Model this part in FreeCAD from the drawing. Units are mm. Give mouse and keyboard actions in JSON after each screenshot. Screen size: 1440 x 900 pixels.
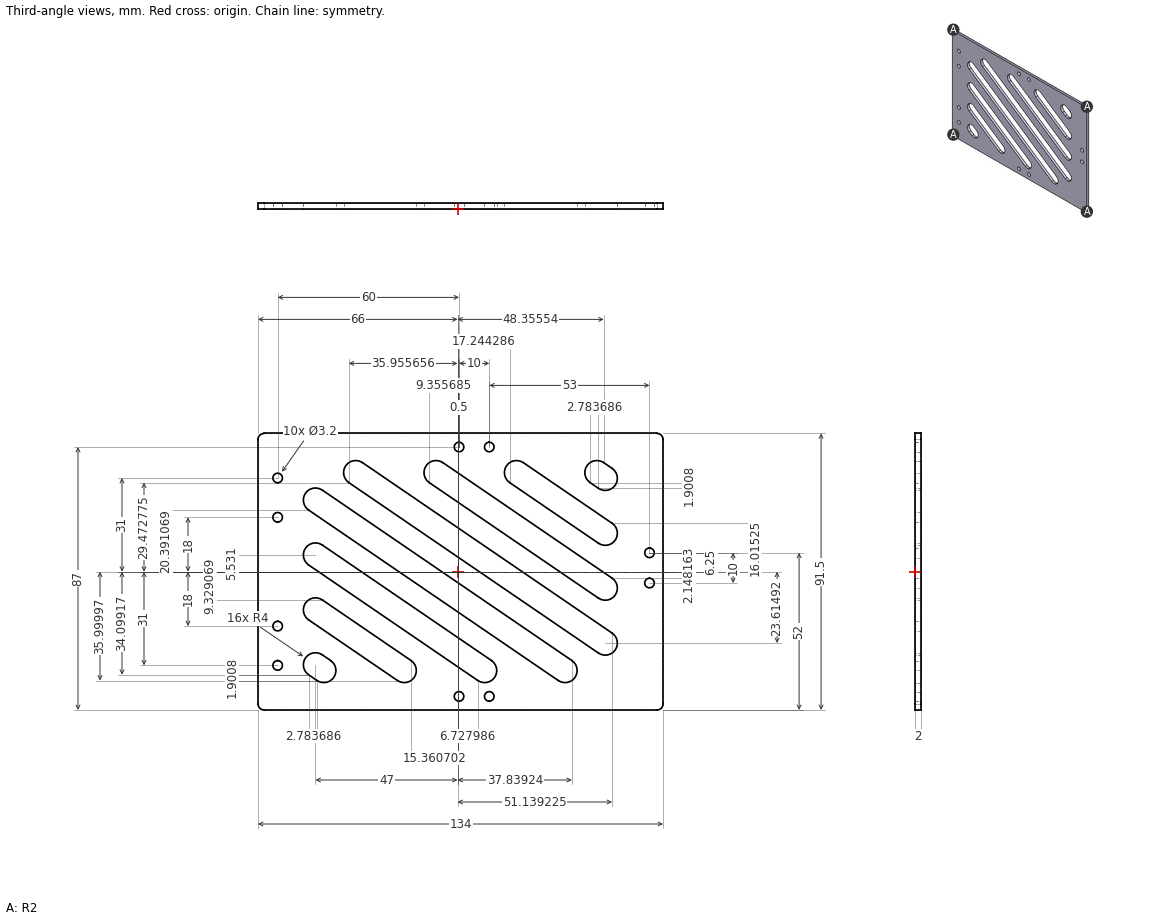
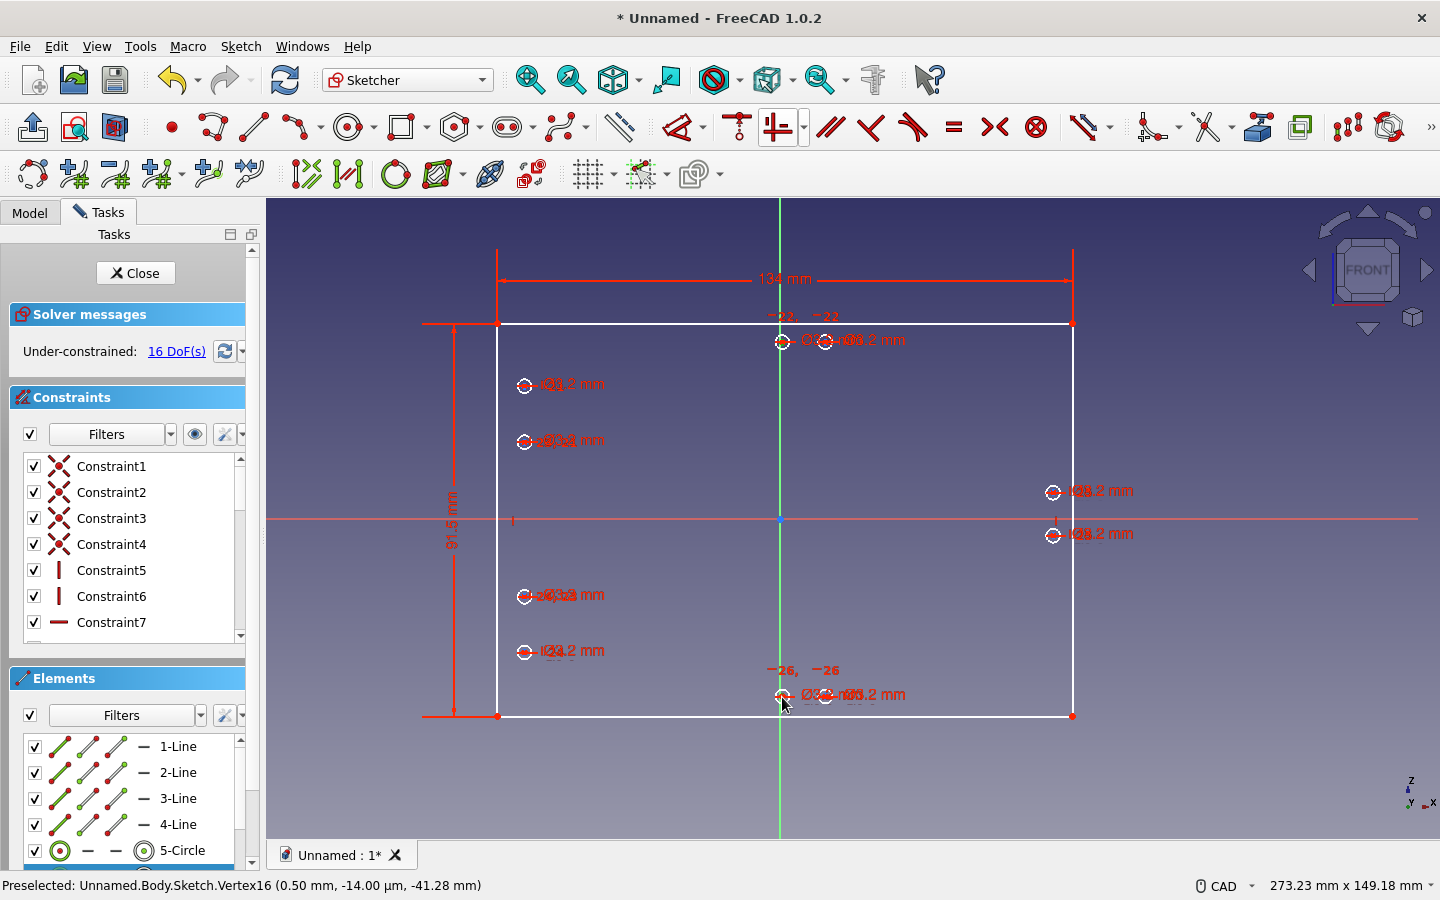
{"action": "left_click", "coordinate": [364, 519]}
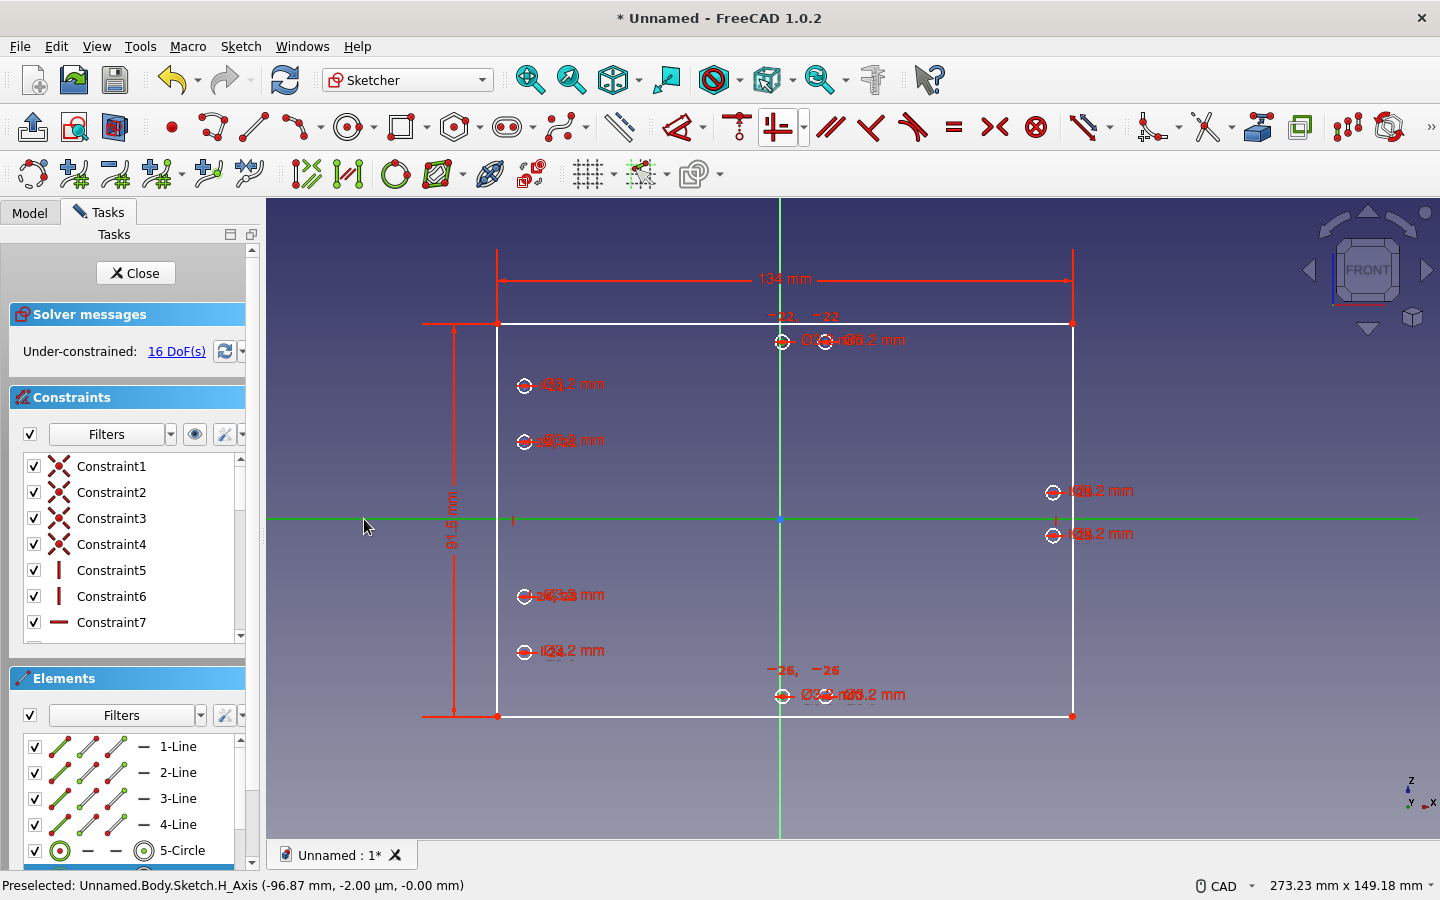
{"action": "left_click", "coordinate": [995, 128]}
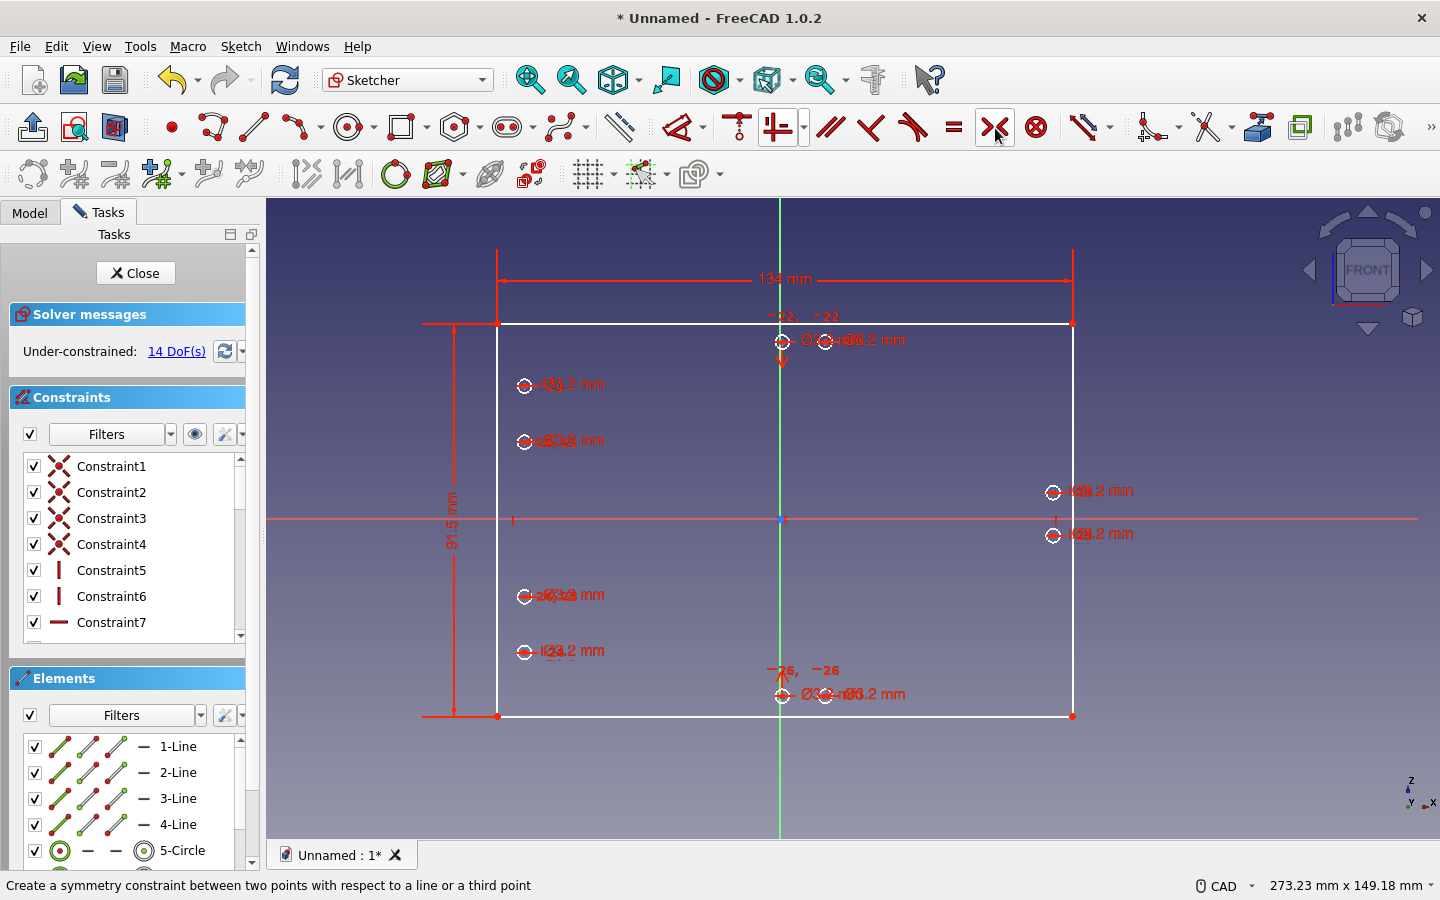
{"action": "left_click", "coordinate": [676, 128]}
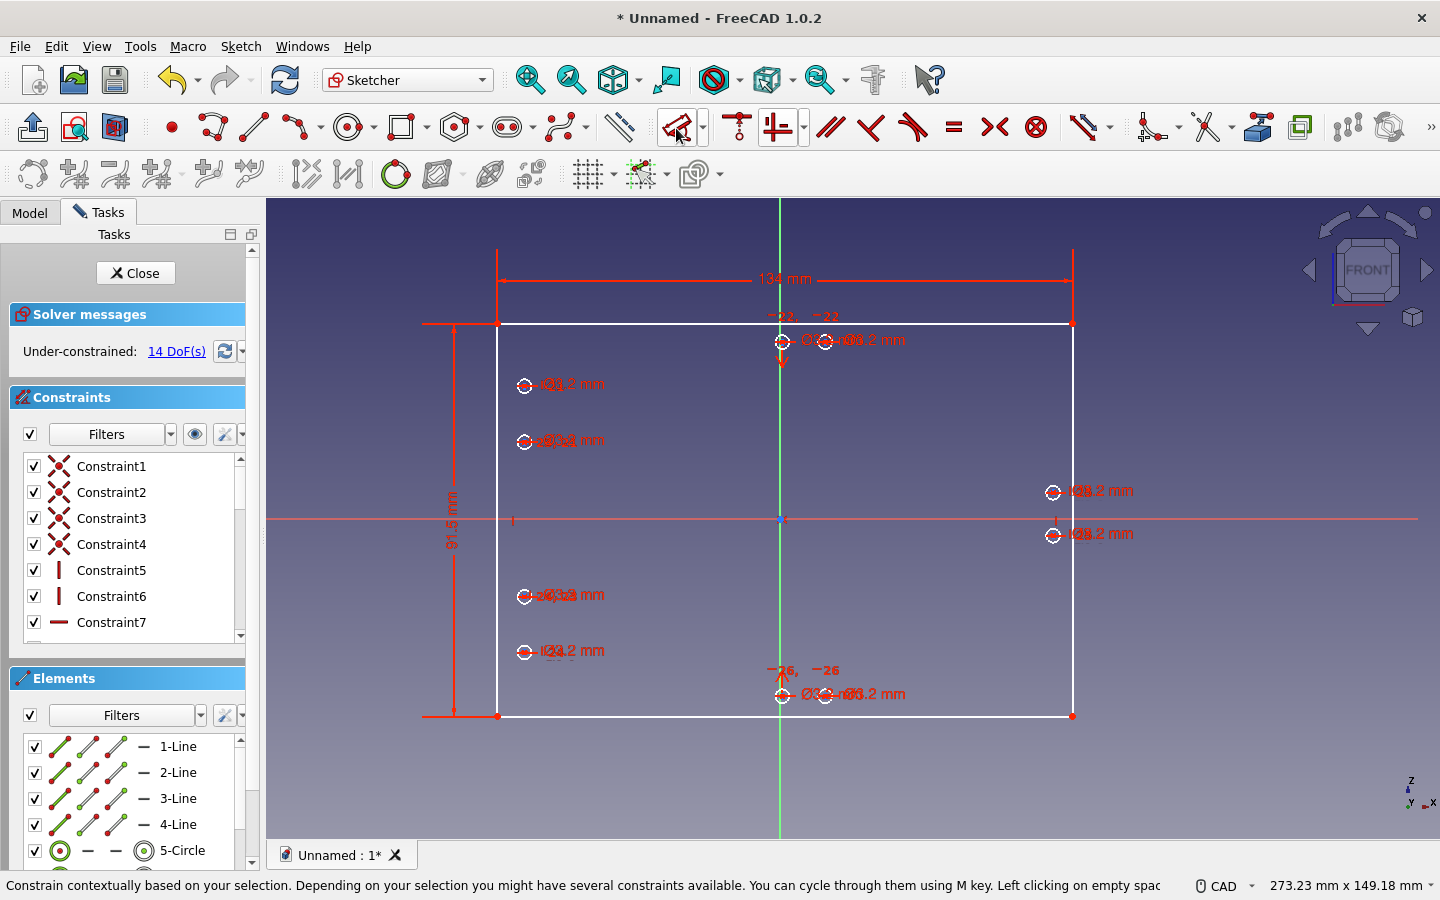
{"action": "left_click", "coordinate": [525, 386]}
{"action": "left_click", "coordinate": [814, 453]}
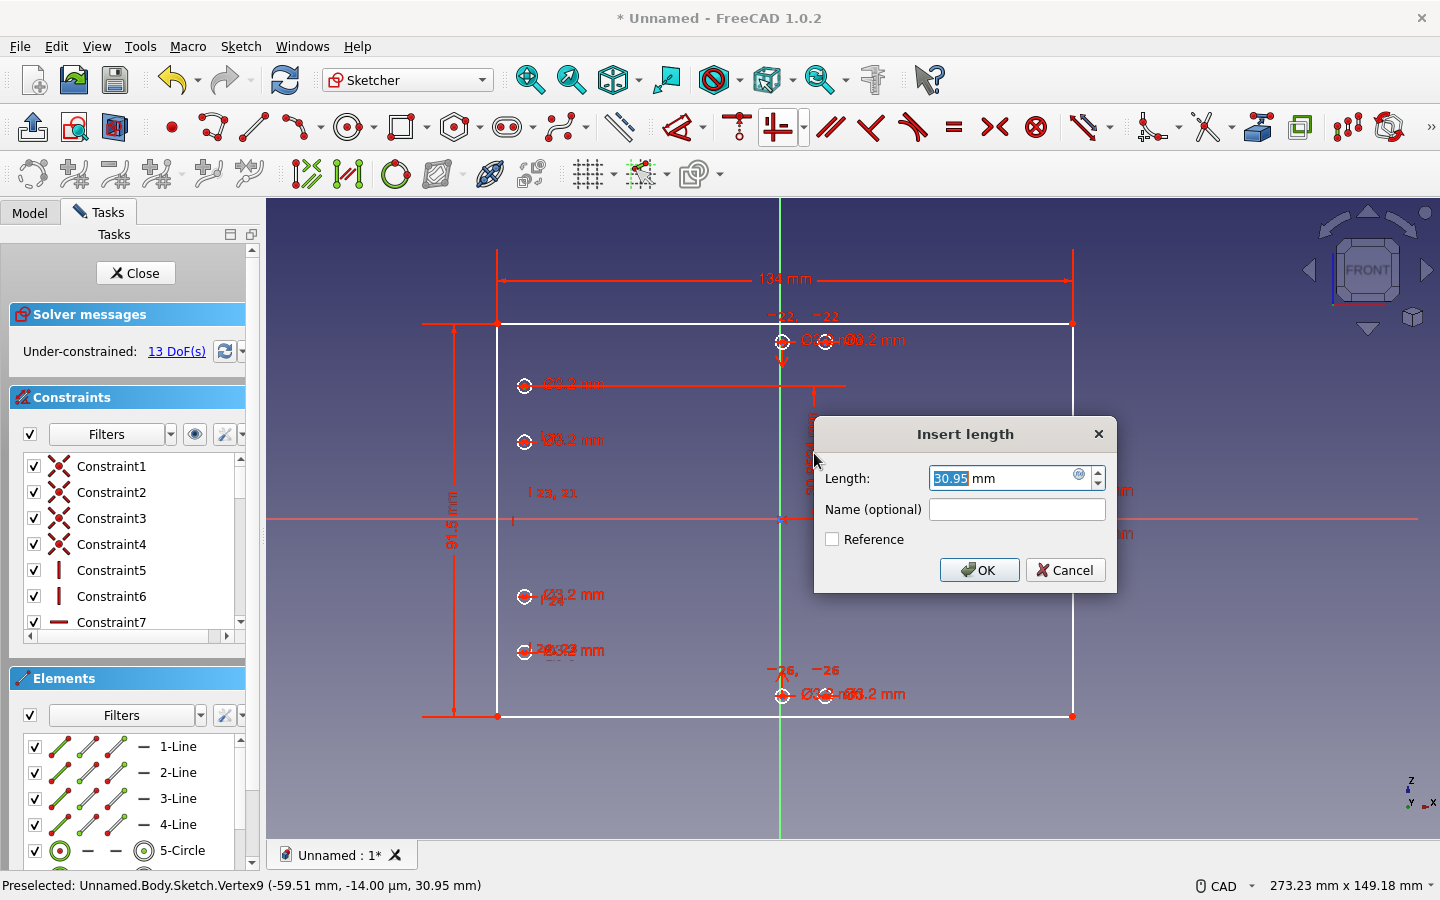
{"action": "type", "text": "31"}
{"action": "key", "text": "Return"}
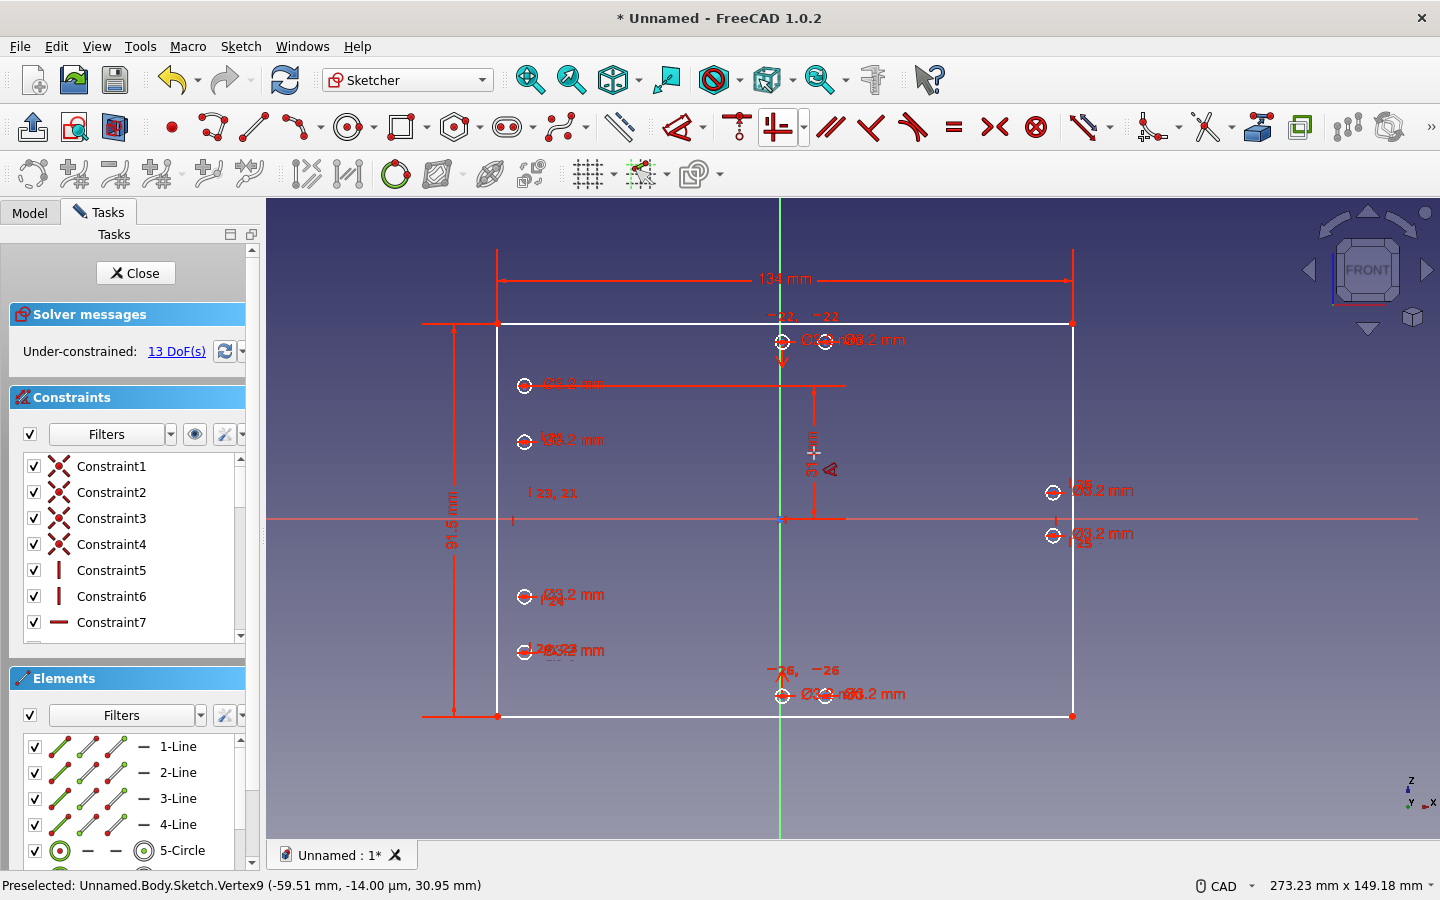
{"action": "left_click", "coordinate": [525, 442]}
{"action": "left_click", "coordinate": [814, 481]}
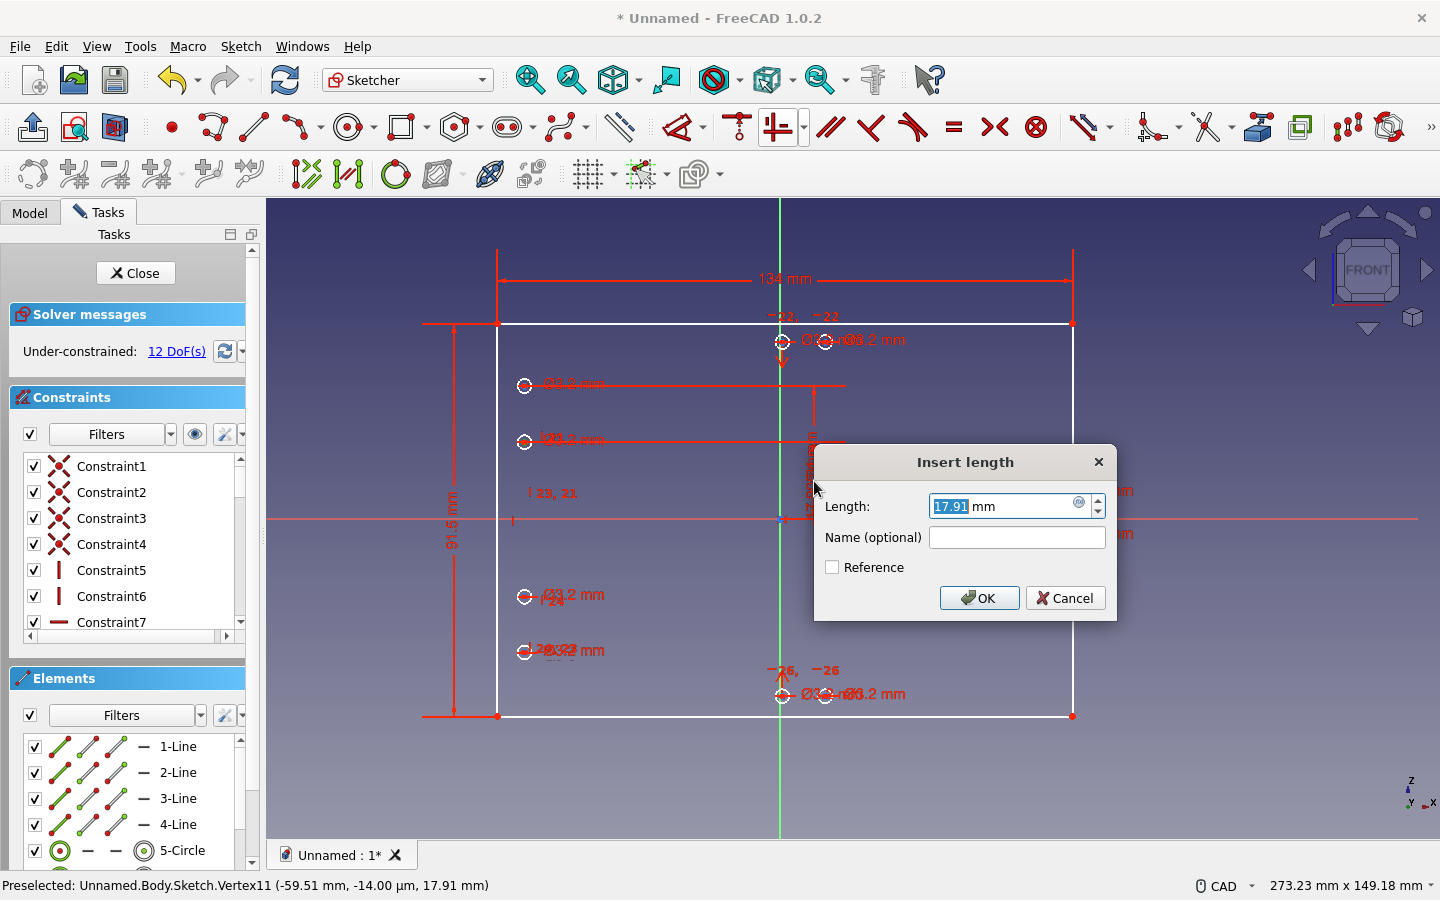
{"action": "type", "text": "18"}
{"action": "key", "text": "Return"}